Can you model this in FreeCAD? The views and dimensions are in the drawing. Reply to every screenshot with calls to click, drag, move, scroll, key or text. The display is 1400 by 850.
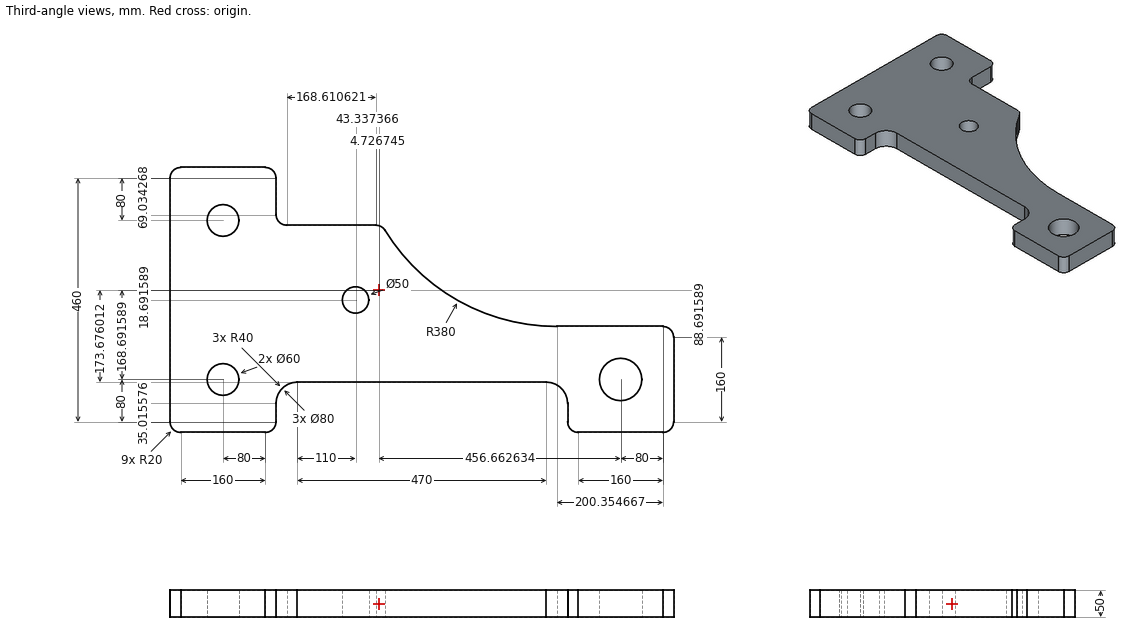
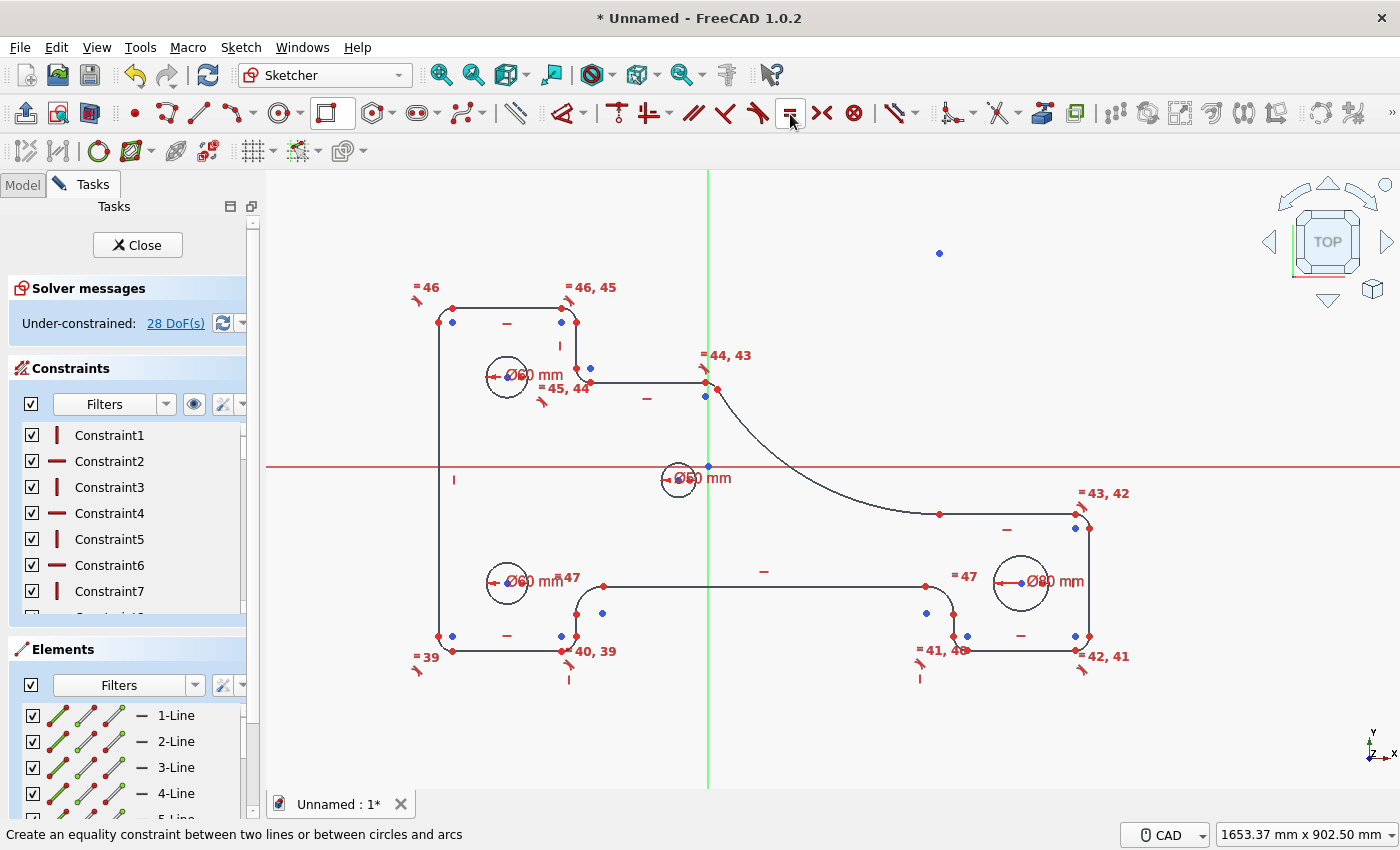
click(562, 114)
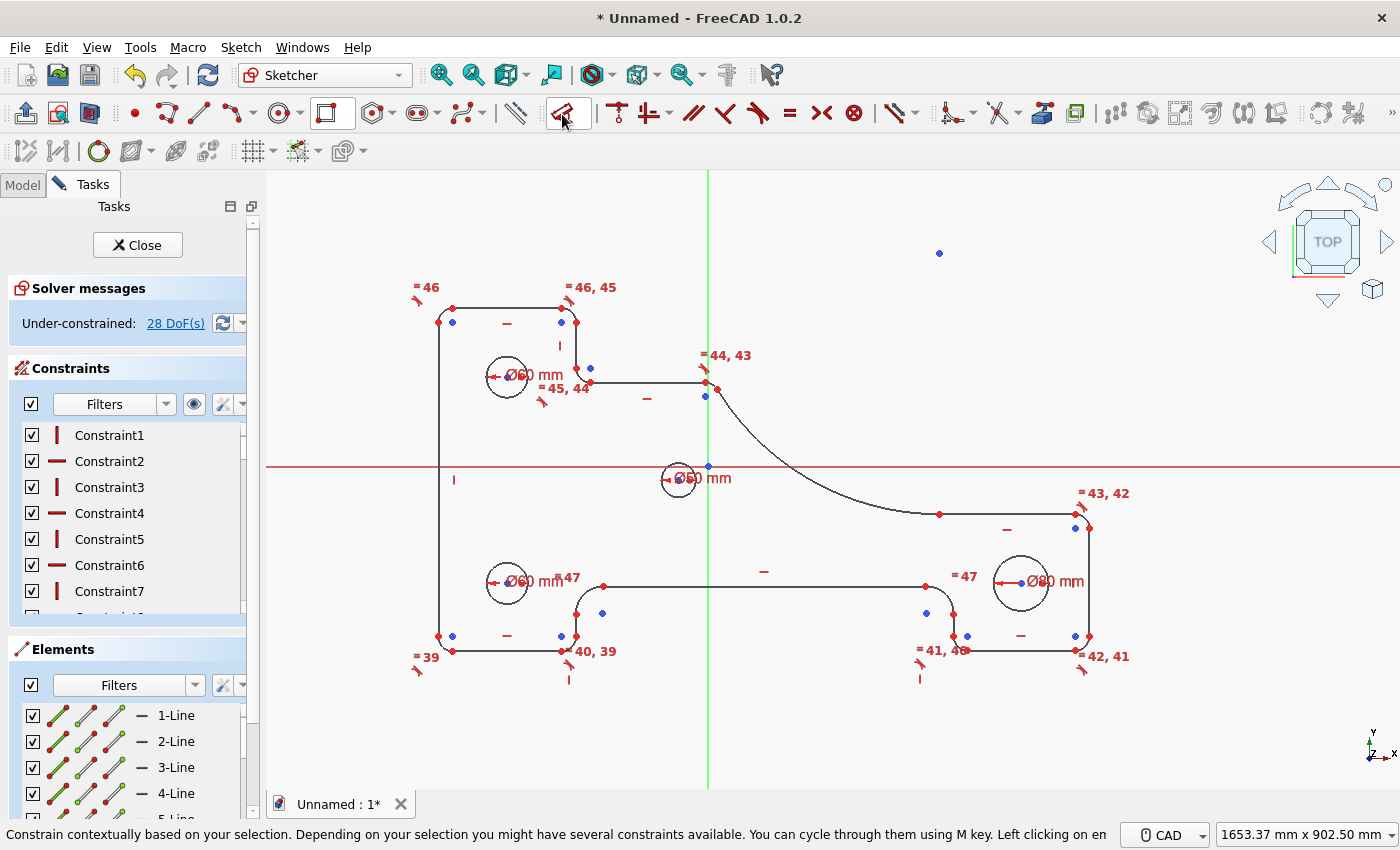
scroll(443, 647, up, 6)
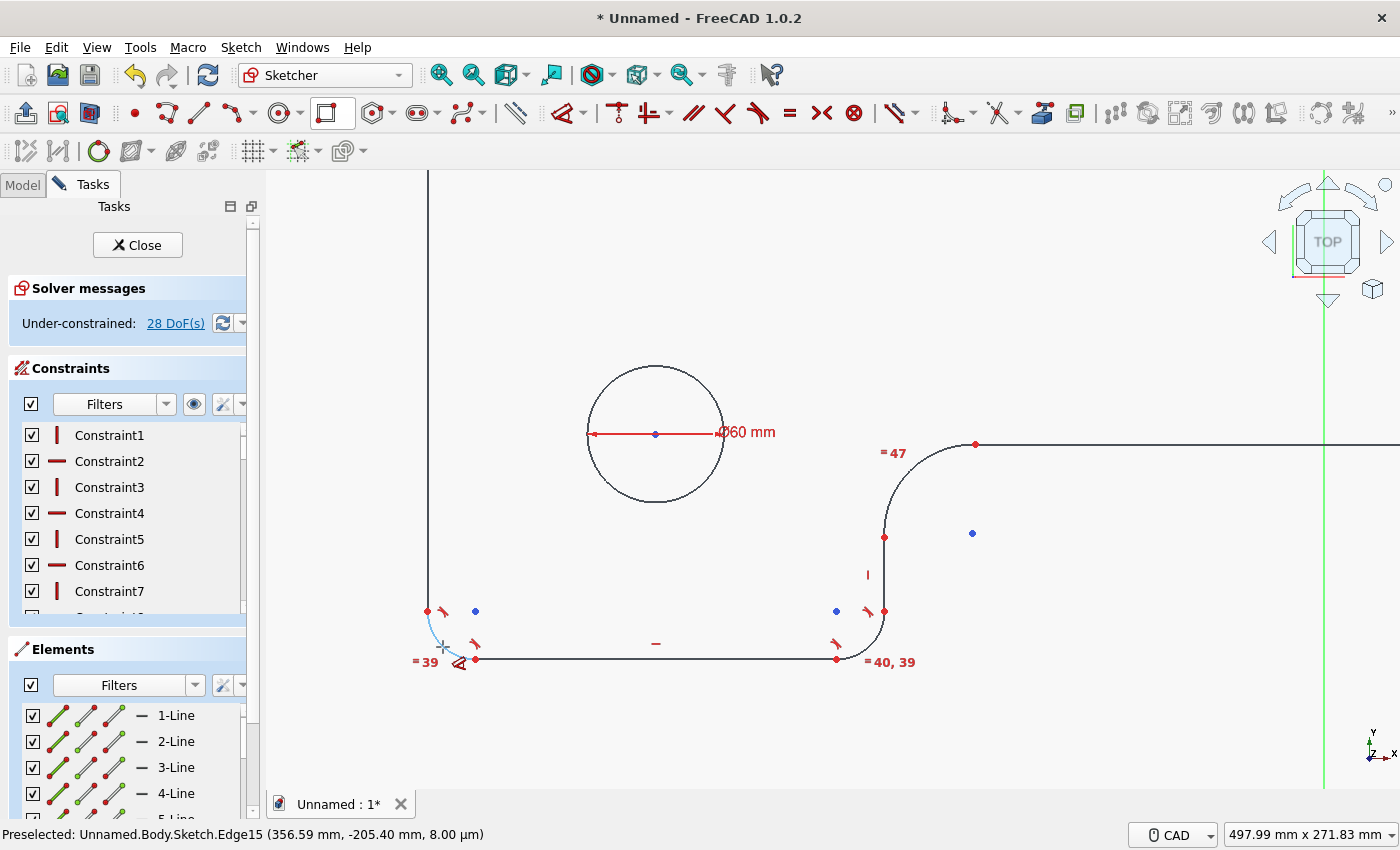
click(442, 645)
click(419, 668)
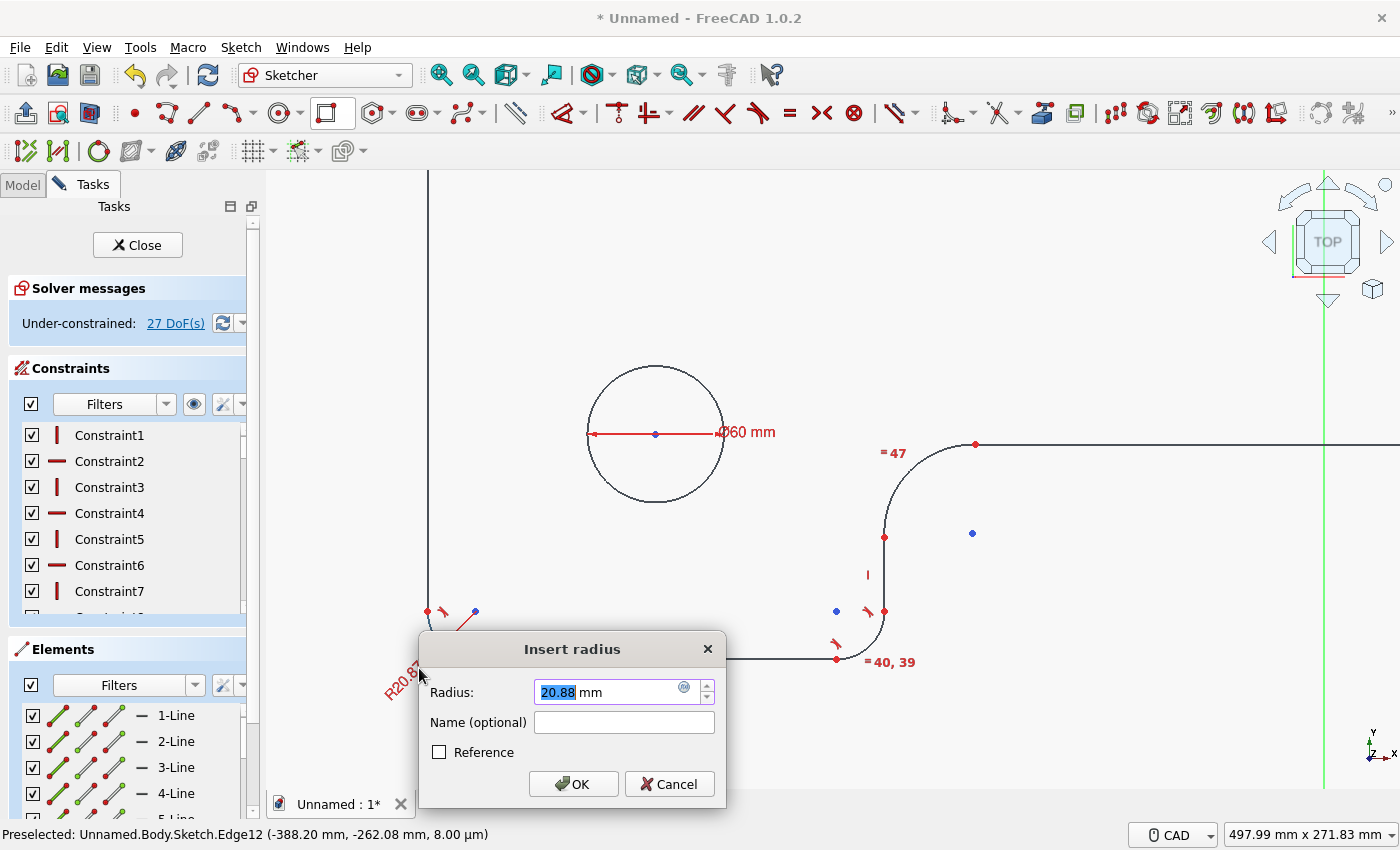
text(20)
key(Return)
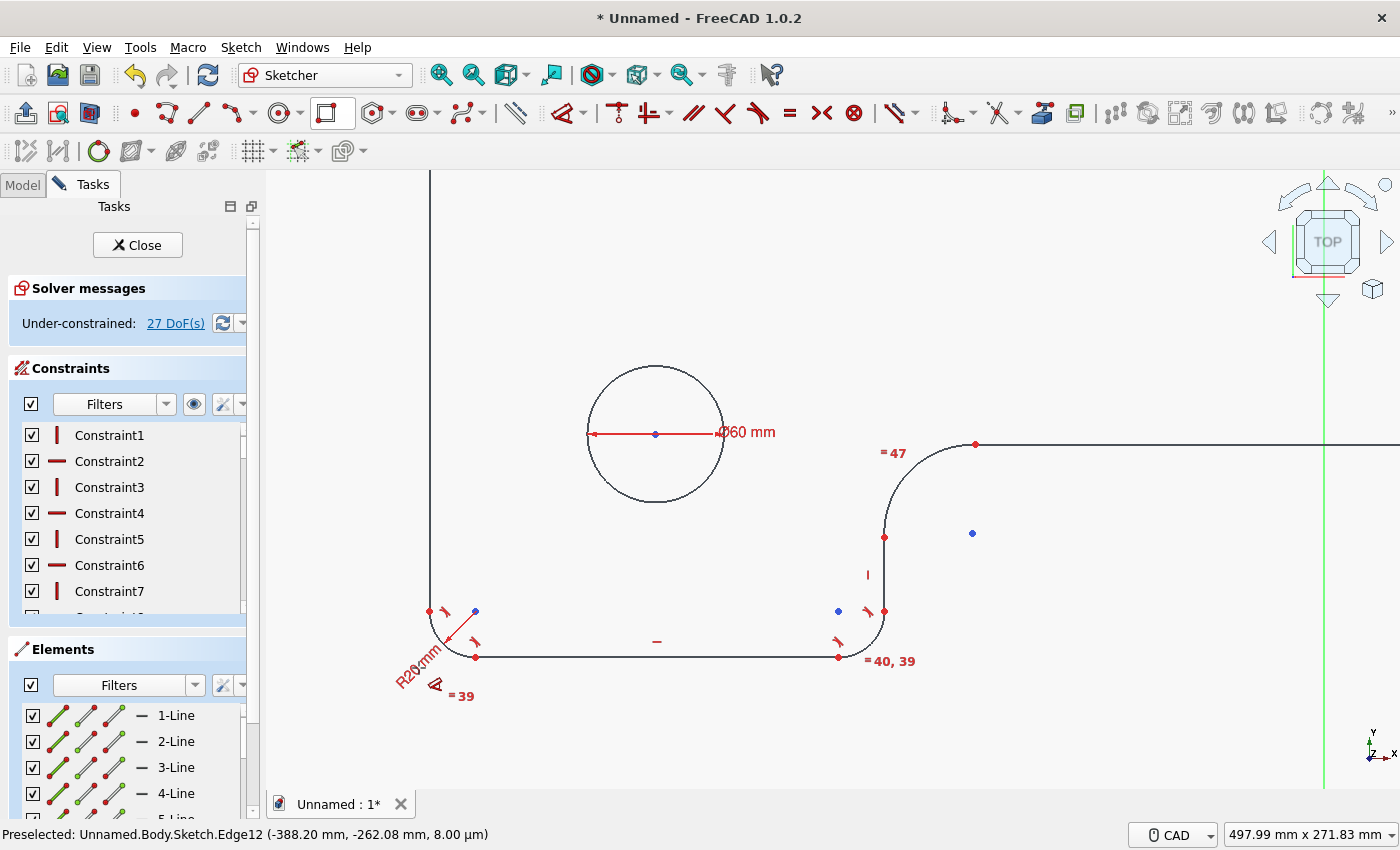
click(933, 454)
click(919, 425)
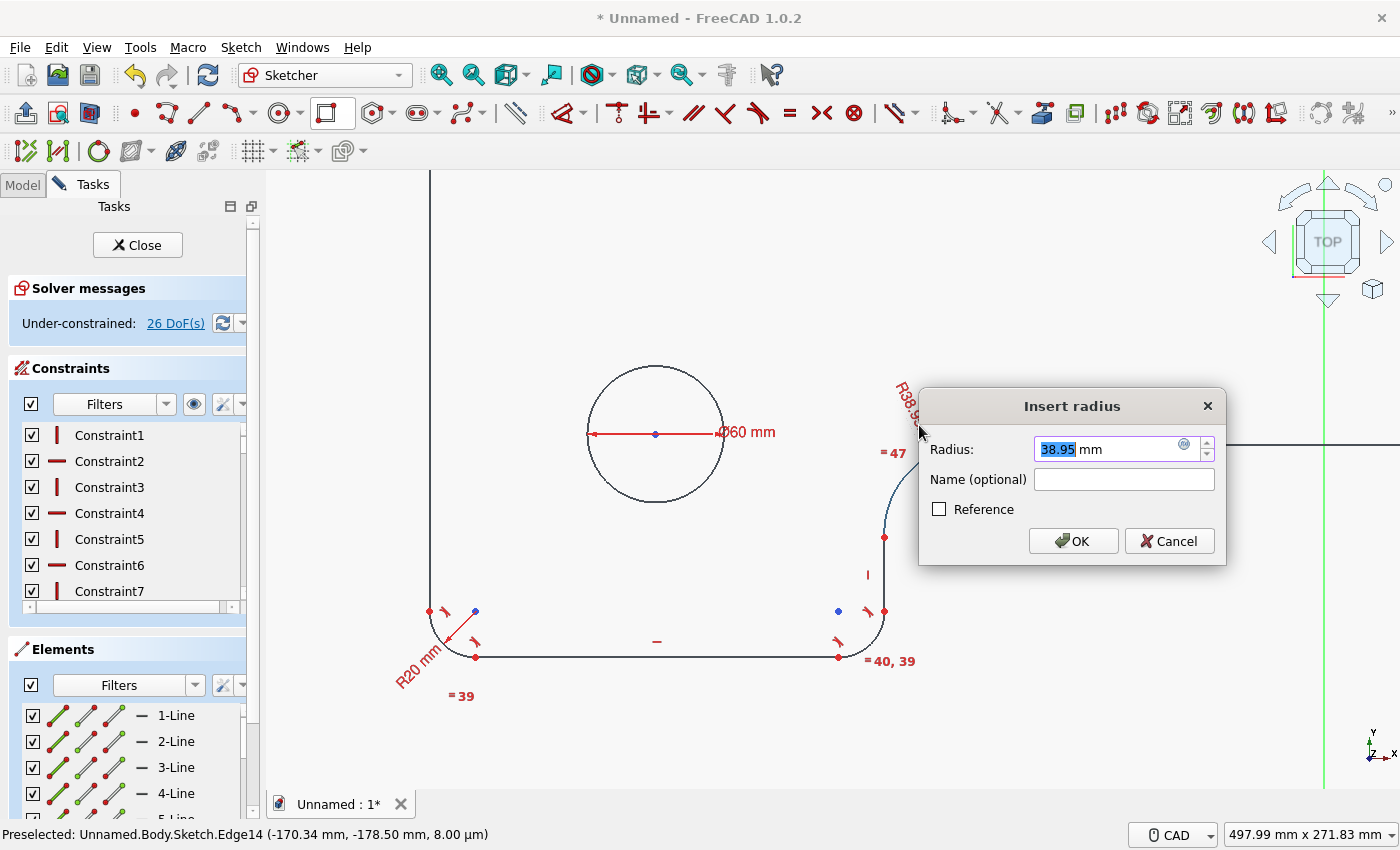
text(40)
key(Return)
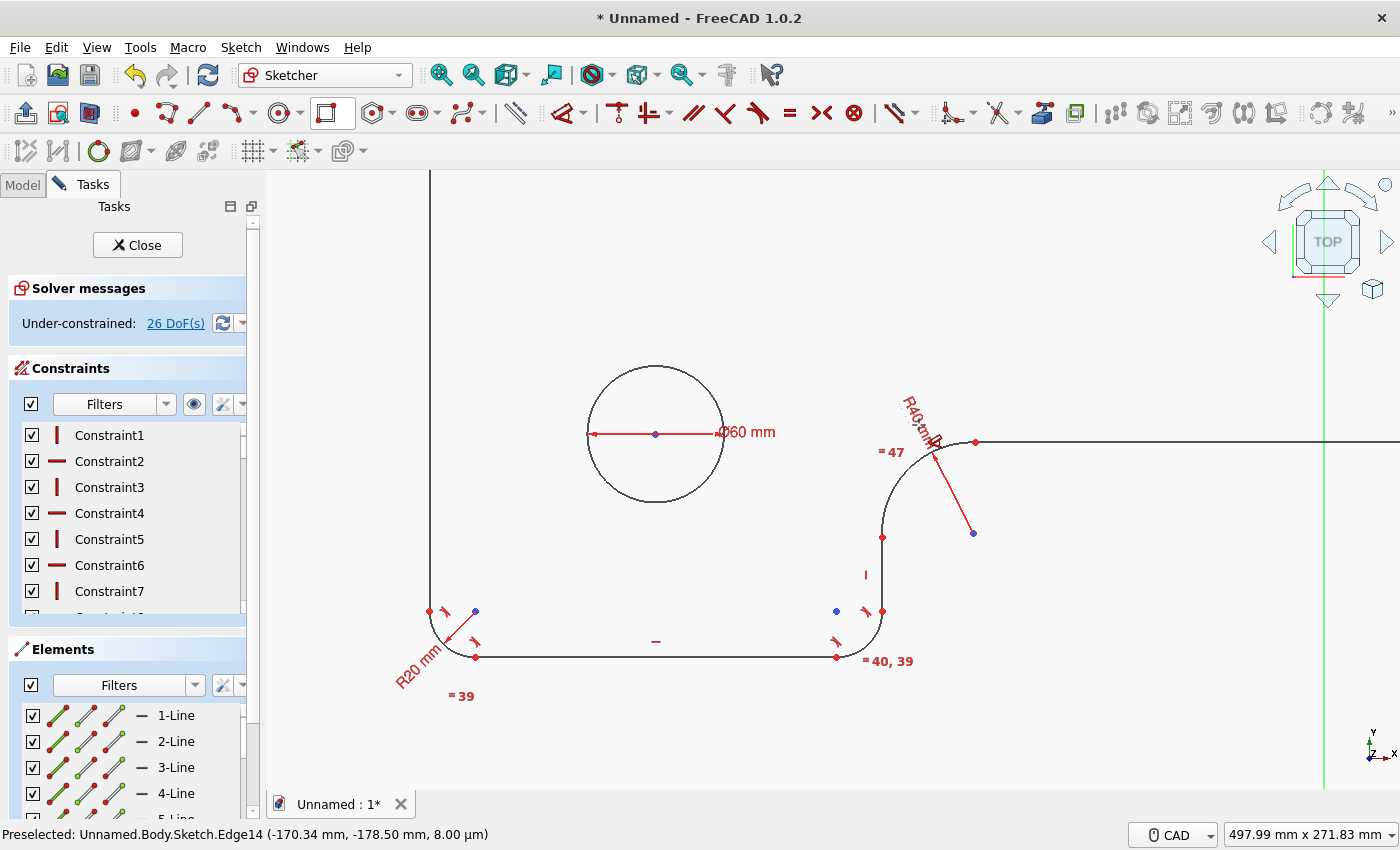
scroll(443, 648, down, 6)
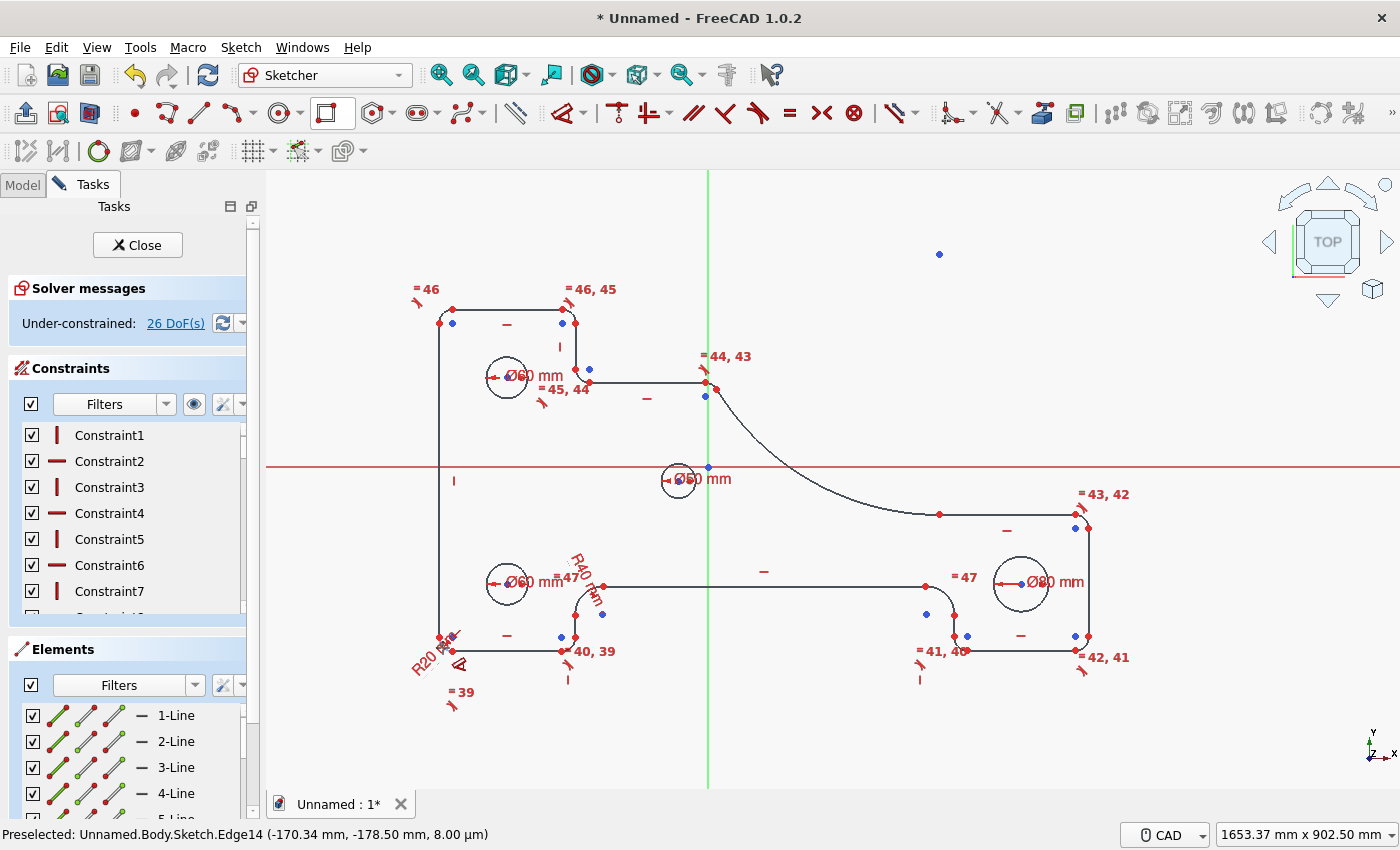
click(768, 451)
click(665, 356)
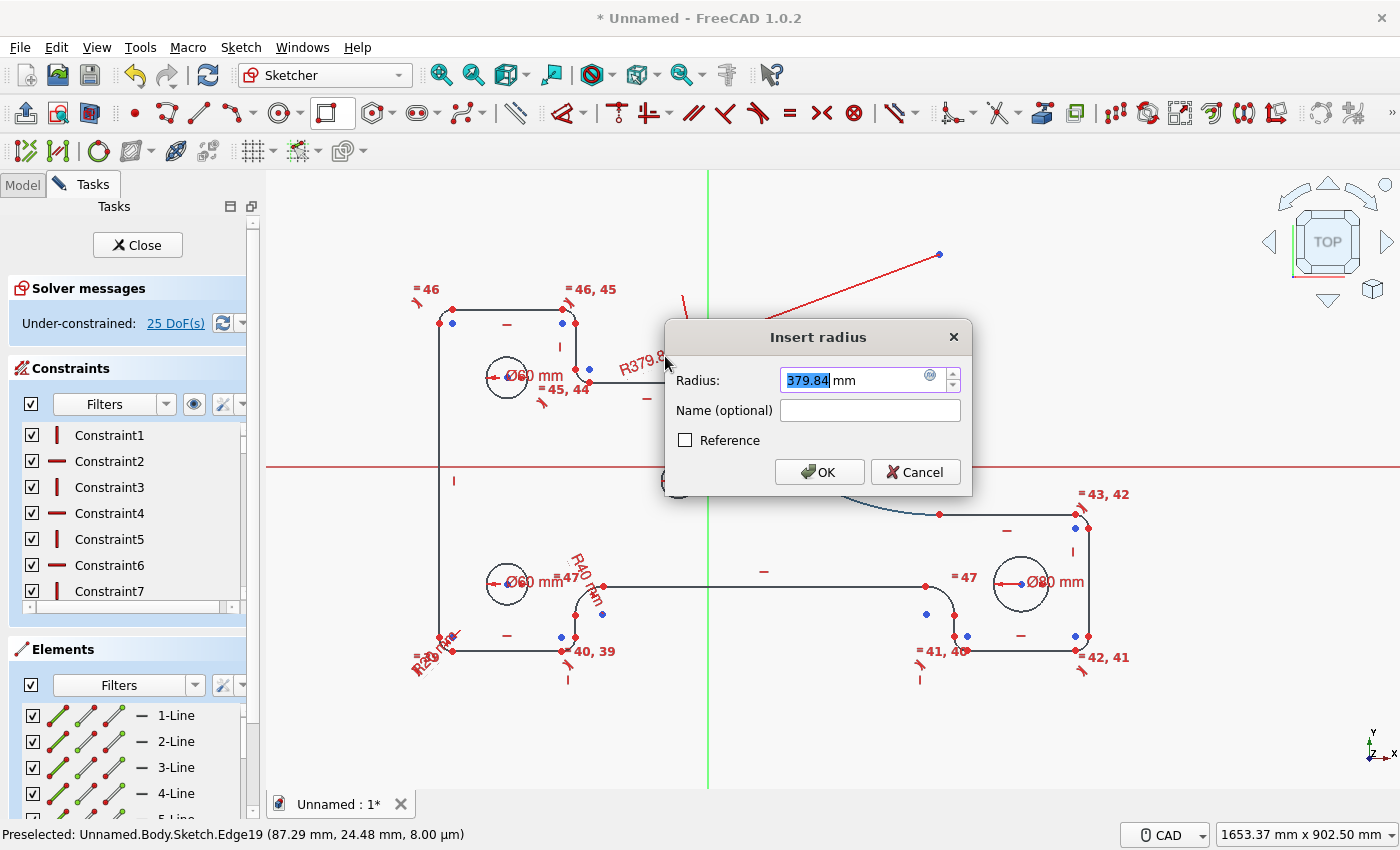
text(380)
key(Return)